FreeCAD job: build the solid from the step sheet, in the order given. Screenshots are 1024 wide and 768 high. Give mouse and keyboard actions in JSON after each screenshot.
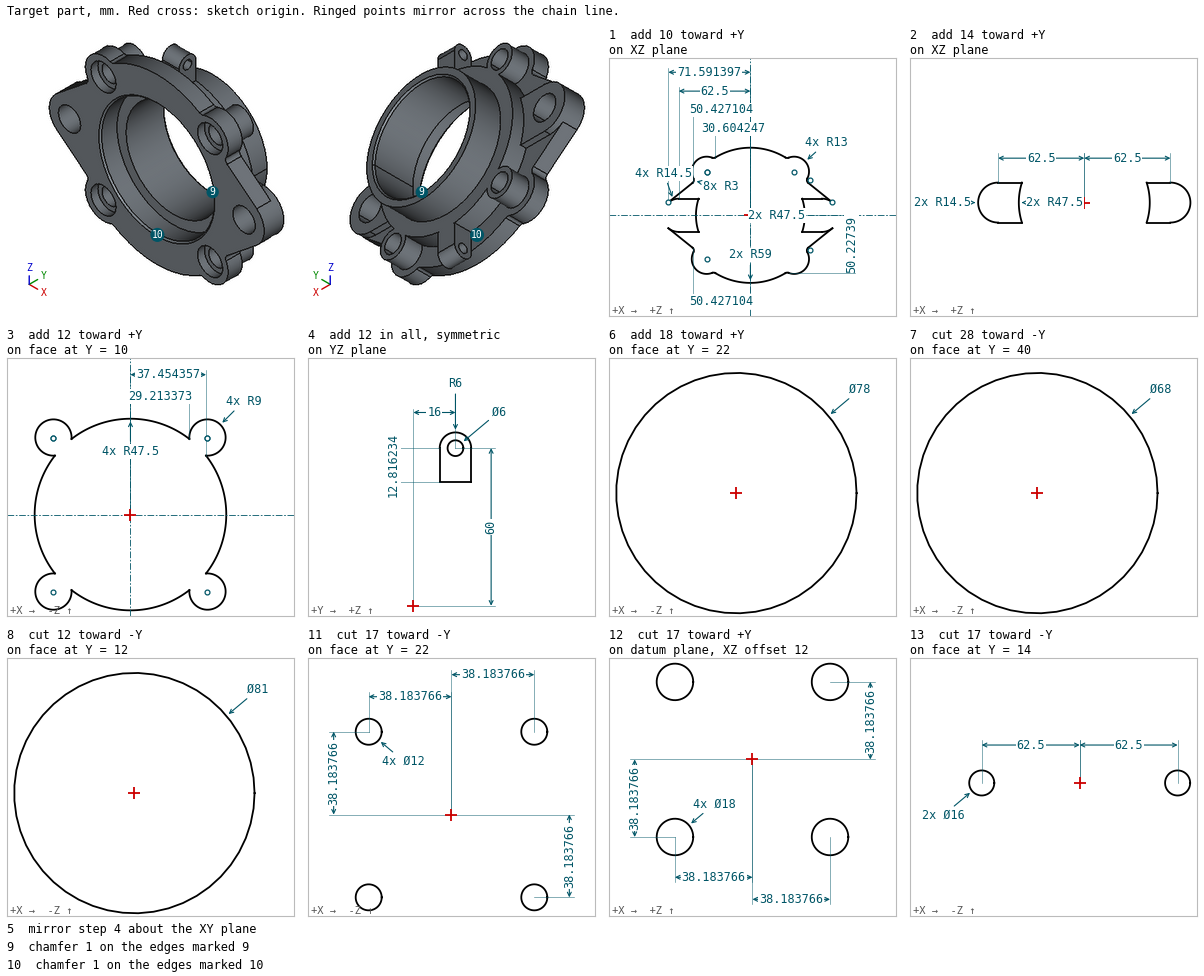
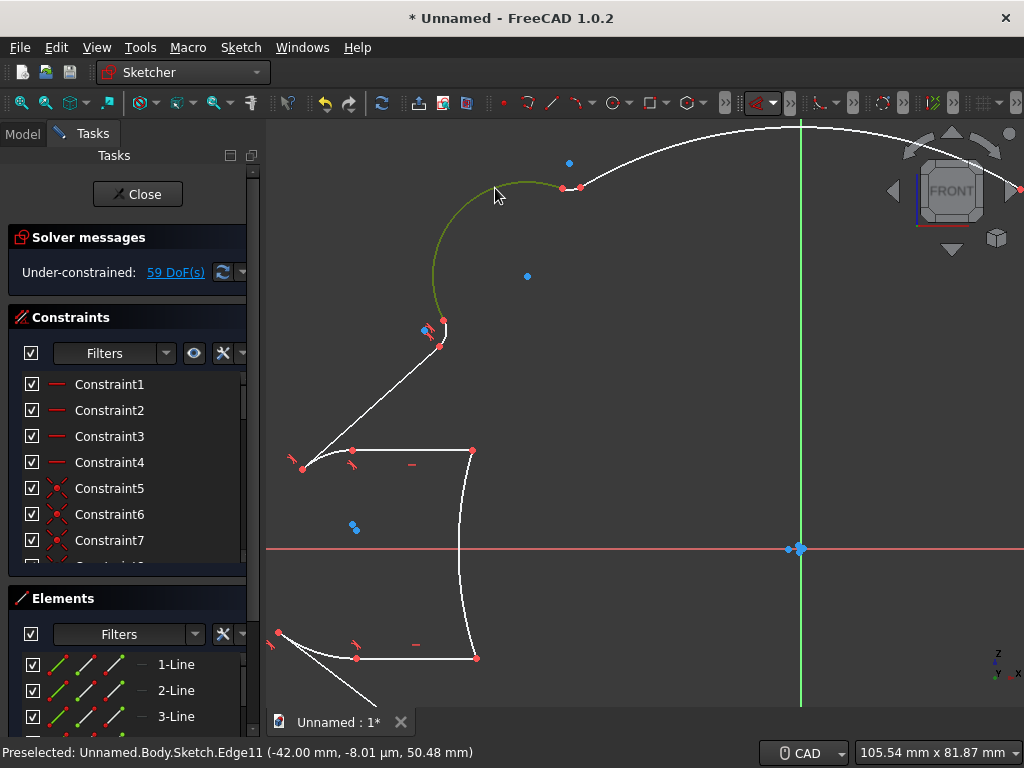
{"action": "scroll", "coordinate": [571, 190], "scroll_direction": "up", "scroll_amount": 2}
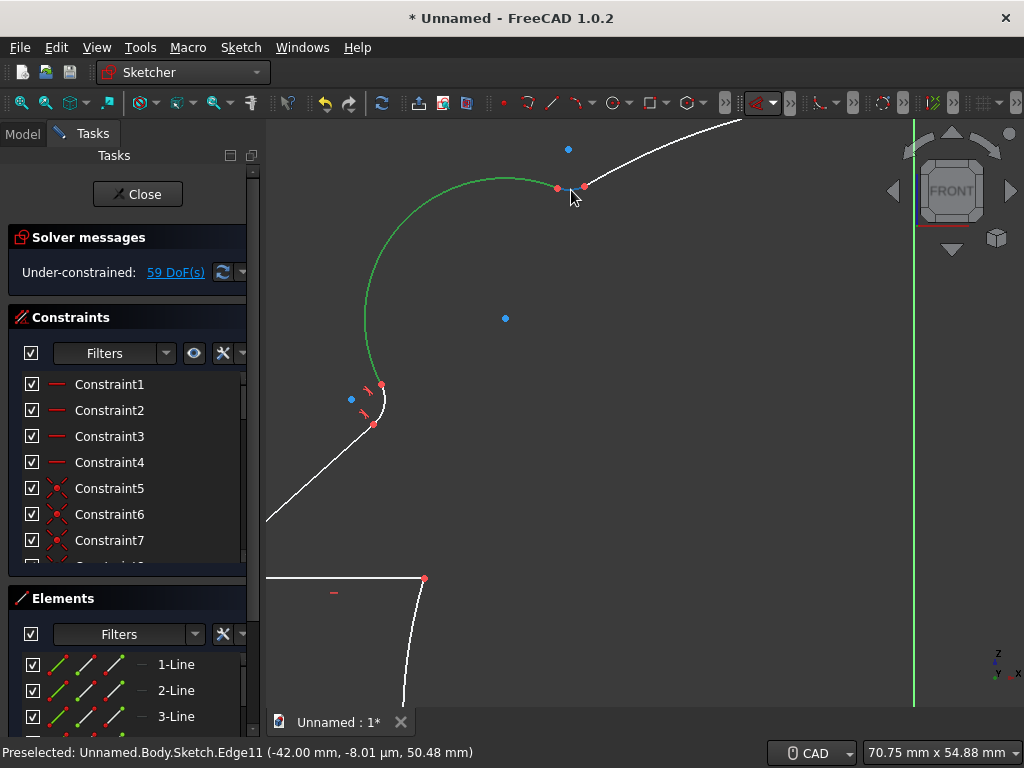
{"action": "left_click", "coordinate": [571, 190]}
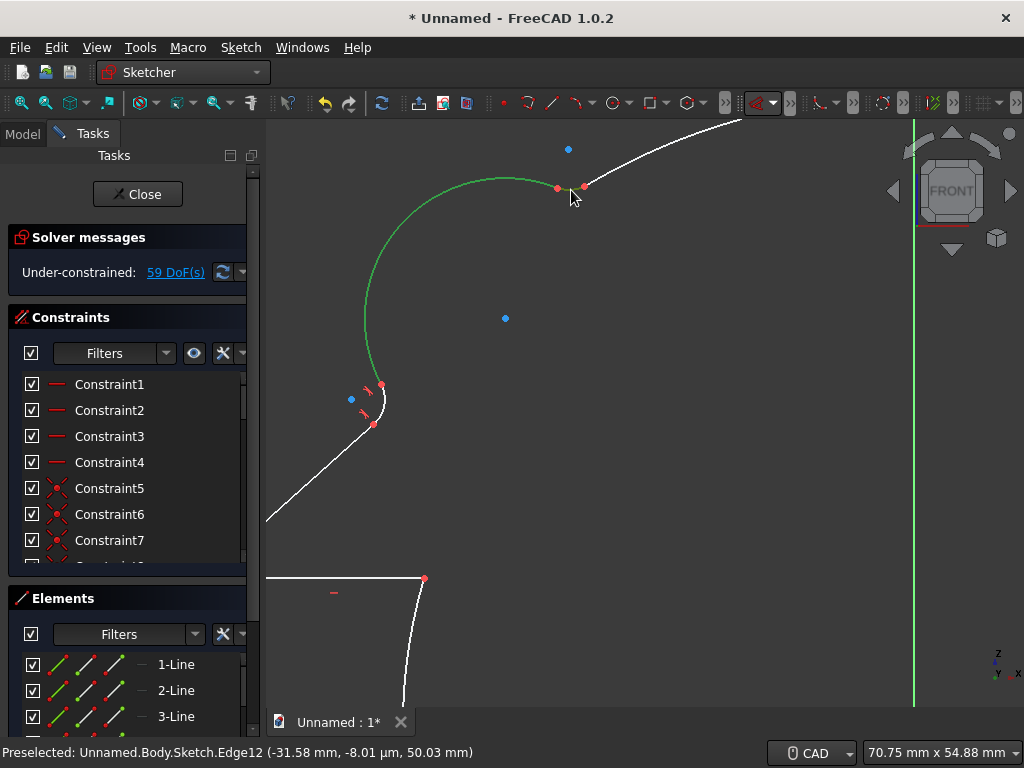
{"action": "key", "text": "t"}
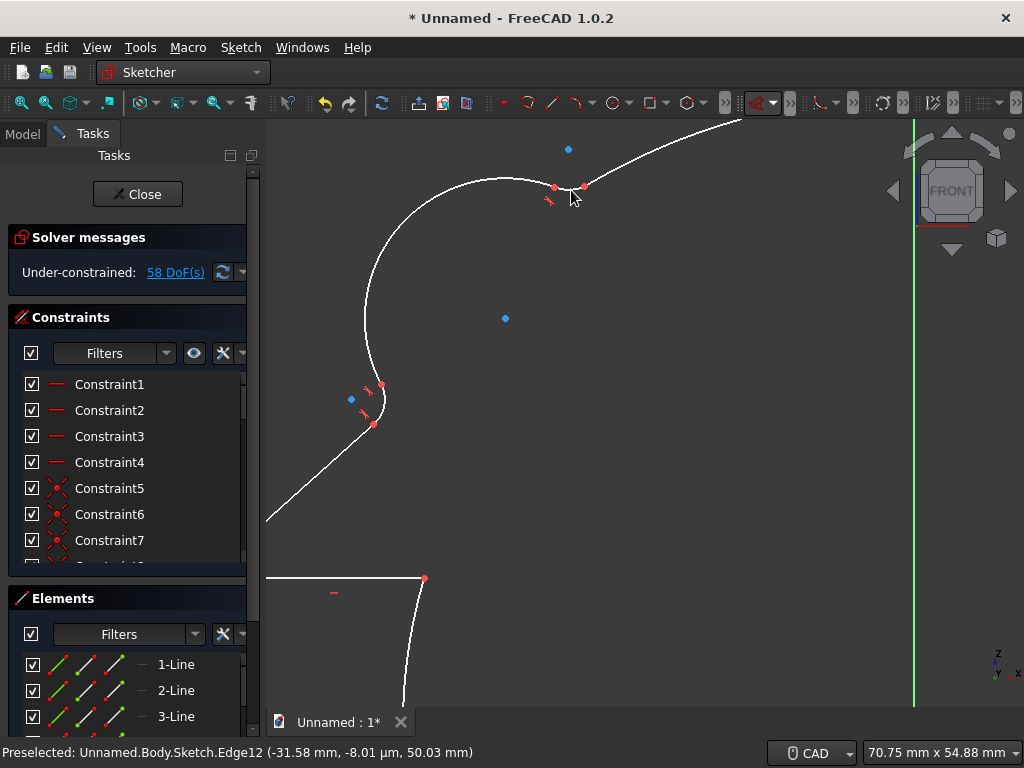
{"action": "scroll", "coordinate": [564, 189], "scroll_direction": "up", "scroll_amount": 3}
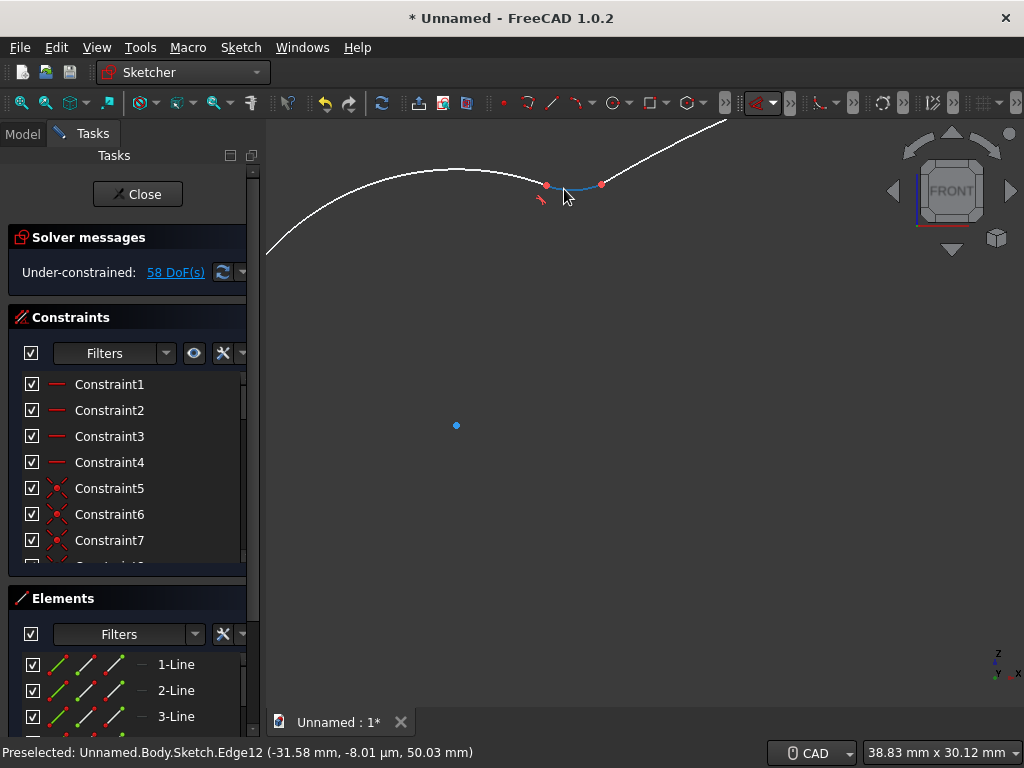
{"action": "left_click", "coordinate": [563, 190]}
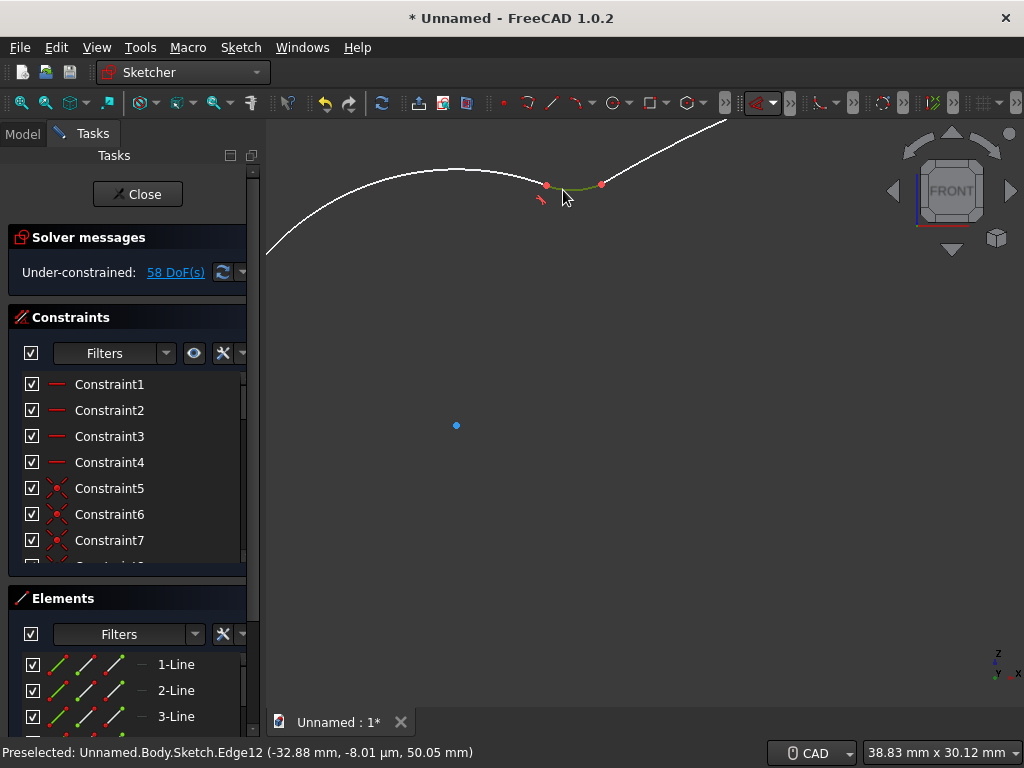
{"action": "scroll", "coordinate": [479, 295], "scroll_direction": "down", "scroll_amount": 10}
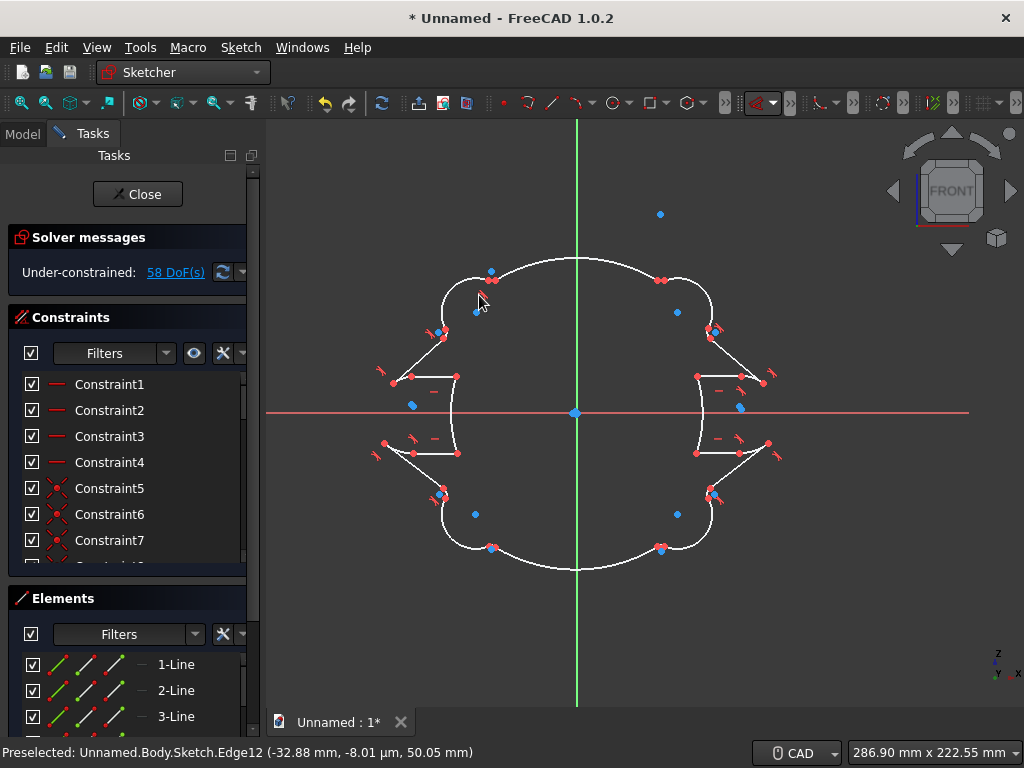
{"action": "left_click", "coordinate": [611, 262]}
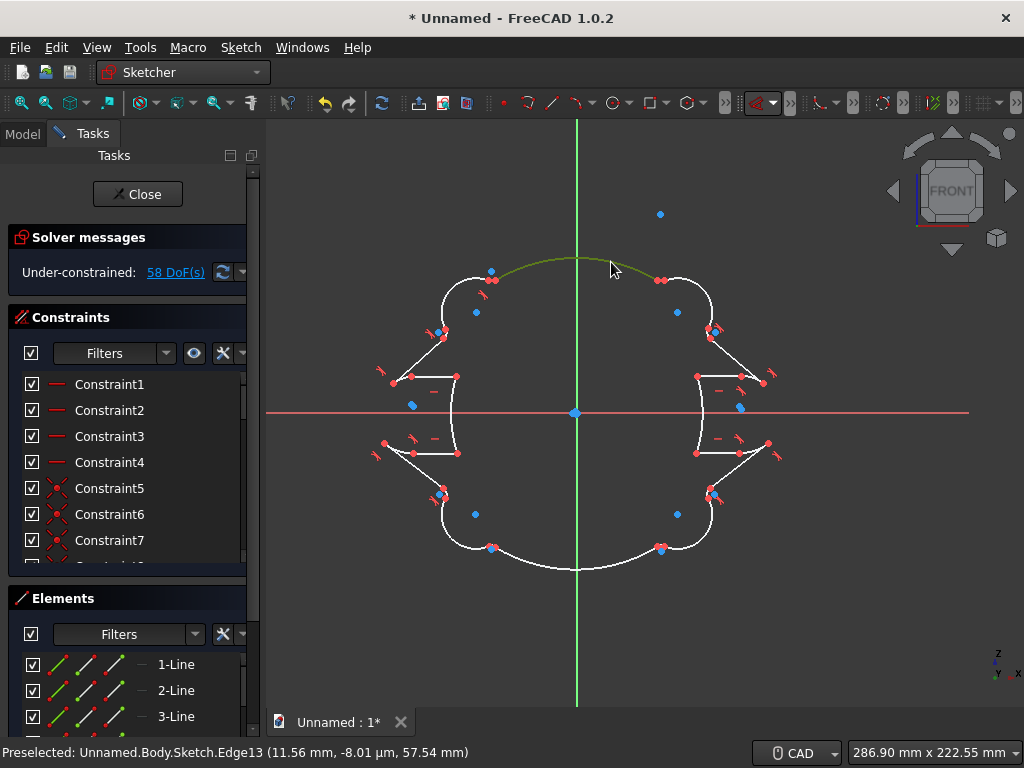
{"action": "key", "text": "t"}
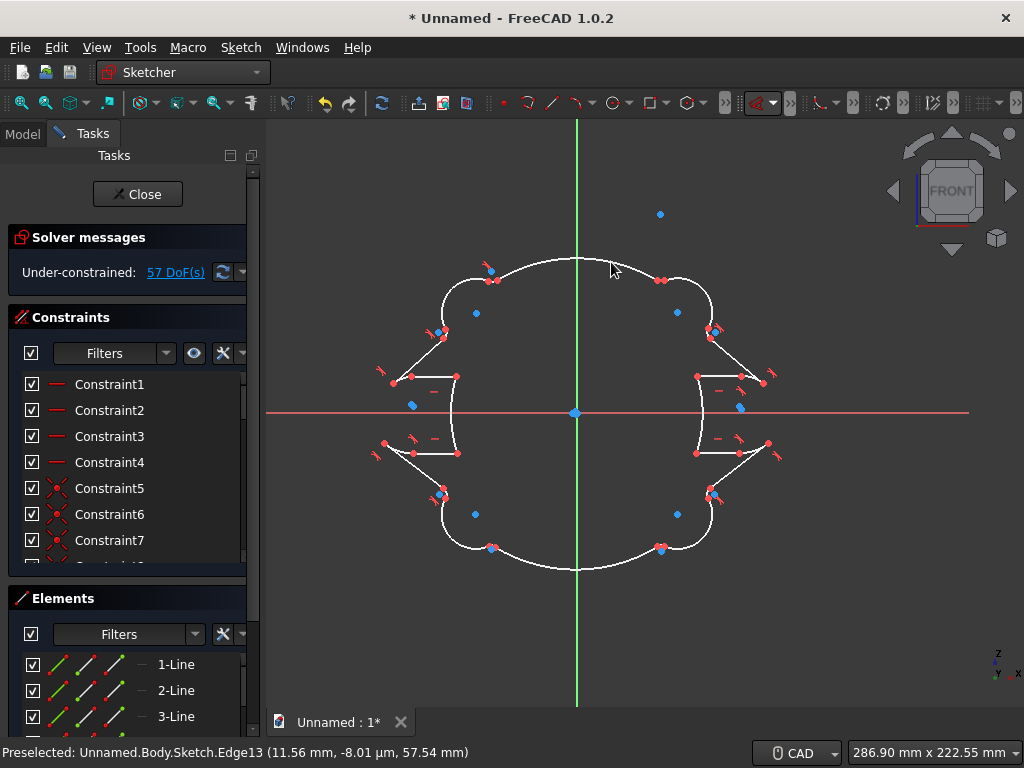
{"action": "left_click", "coordinate": [611, 262]}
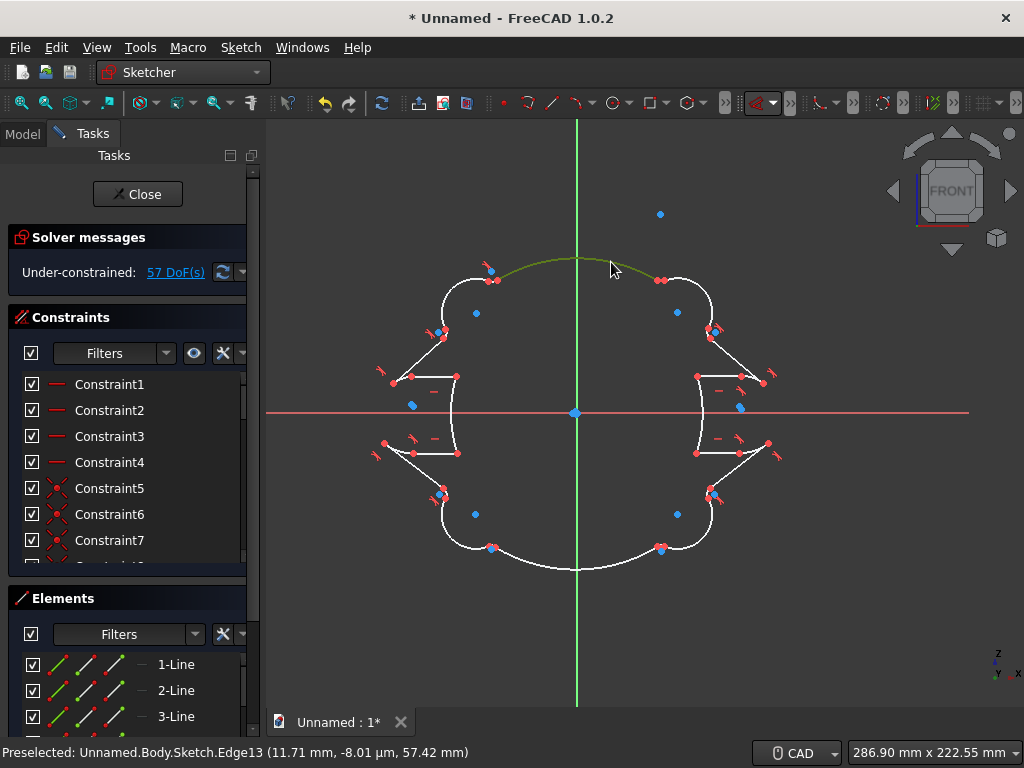
{"action": "scroll", "coordinate": [661, 281], "scroll_direction": "up", "scroll_amount": 7}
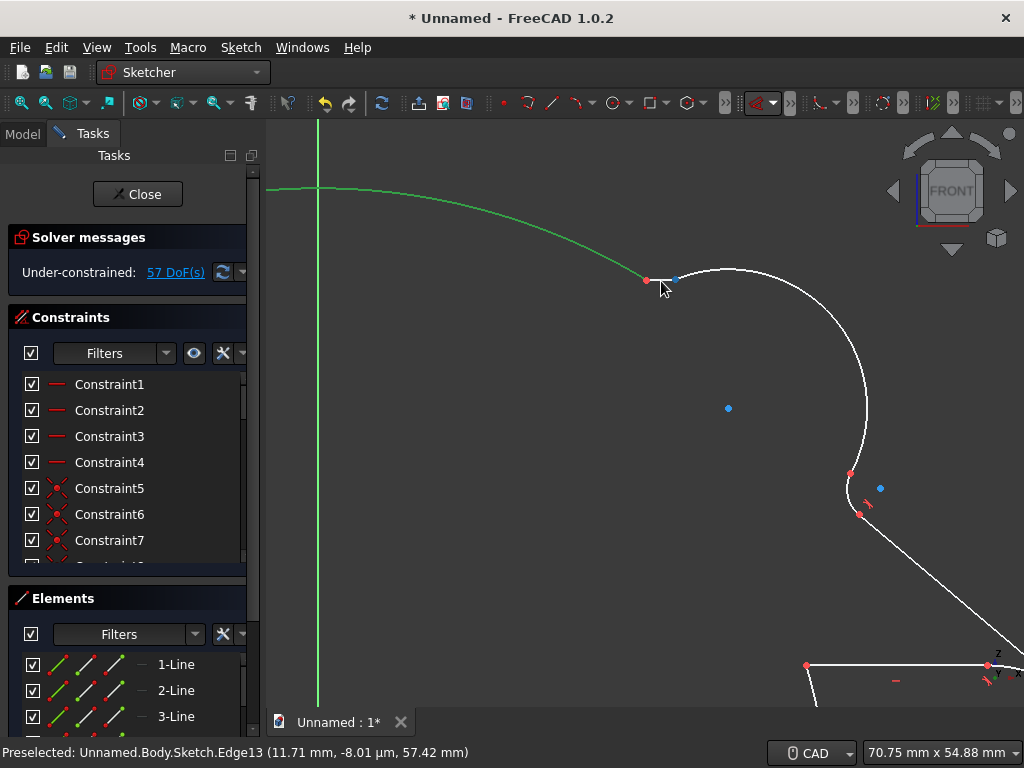
{"action": "left_click", "coordinate": [661, 280]}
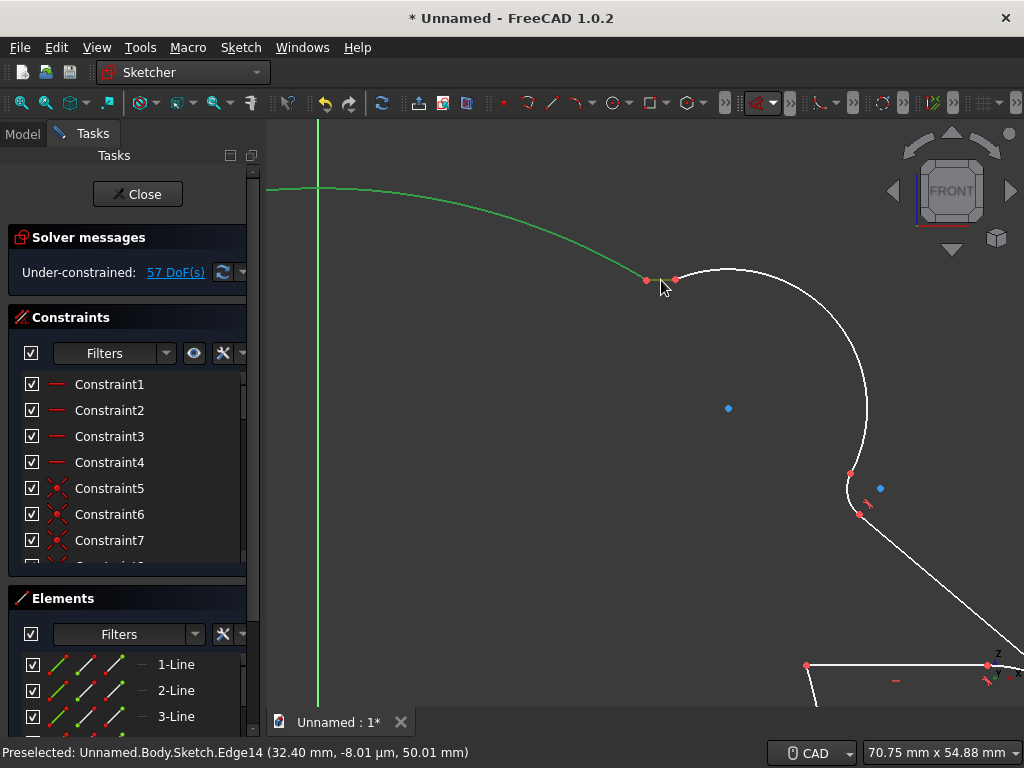
{"action": "key", "text": "t"}